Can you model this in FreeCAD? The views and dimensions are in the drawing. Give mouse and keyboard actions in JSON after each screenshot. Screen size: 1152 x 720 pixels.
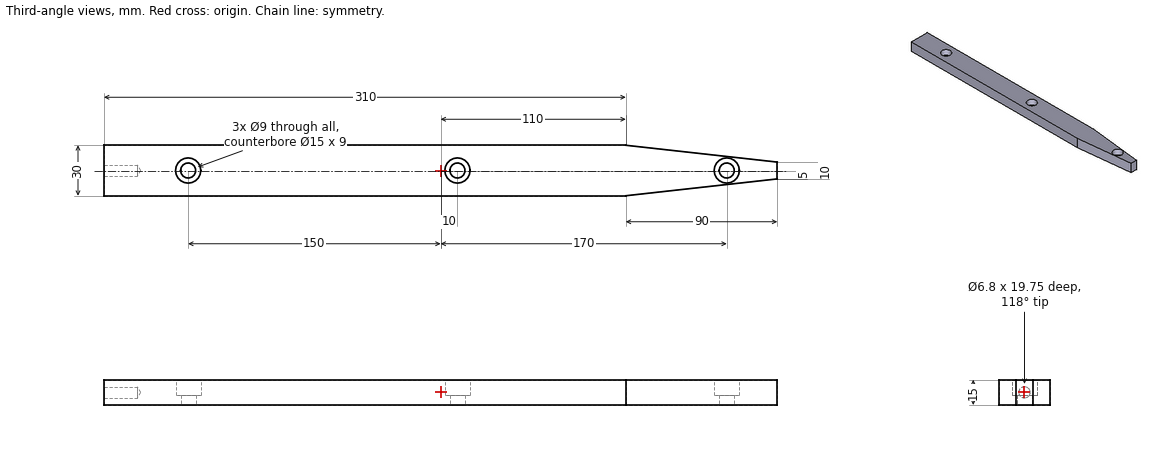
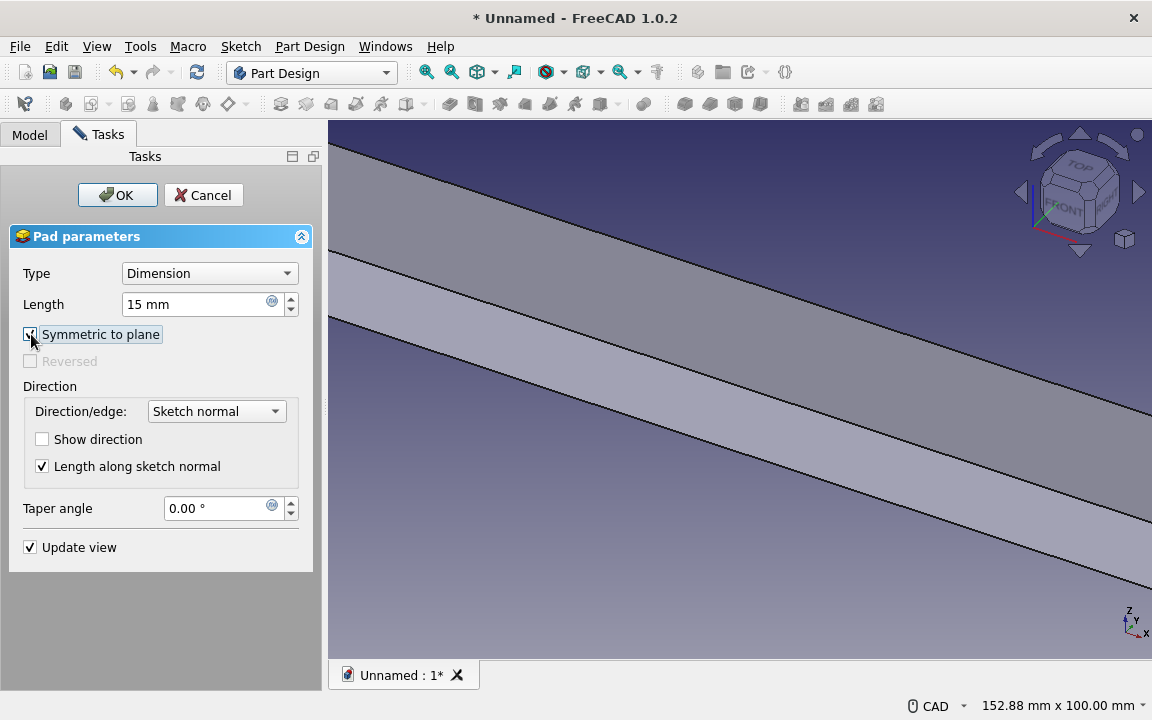
{"action": "left_click", "coordinate": [118, 195]}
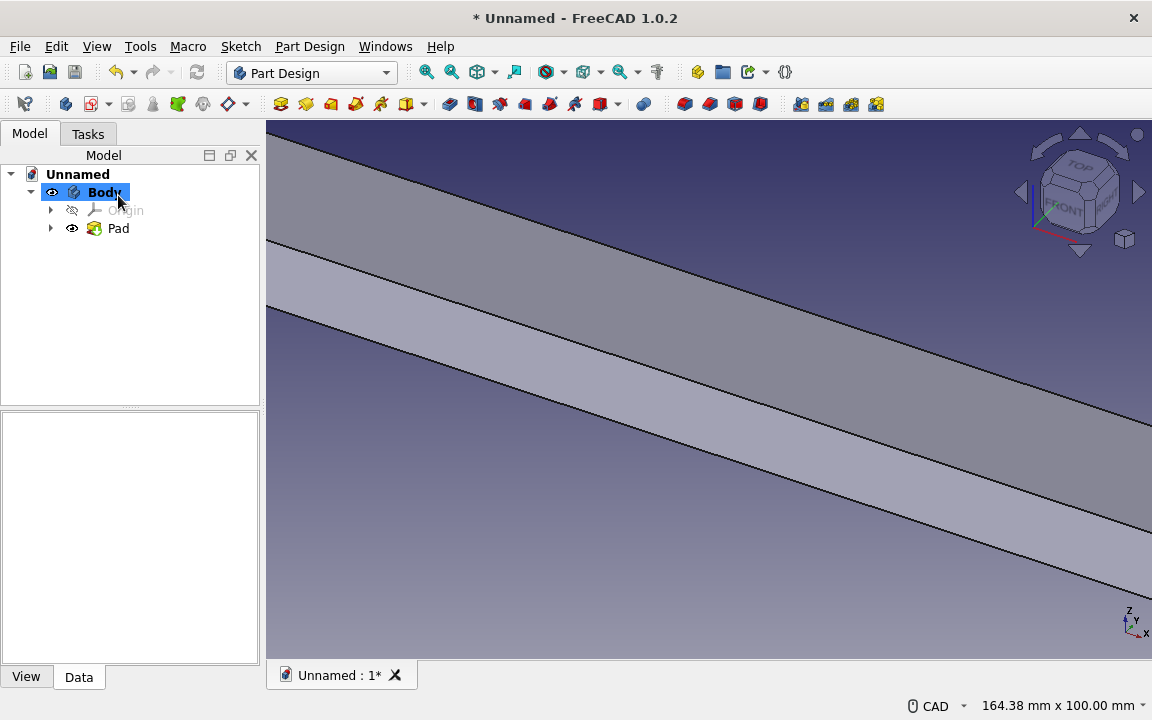
{"action": "key", "text": "v f"}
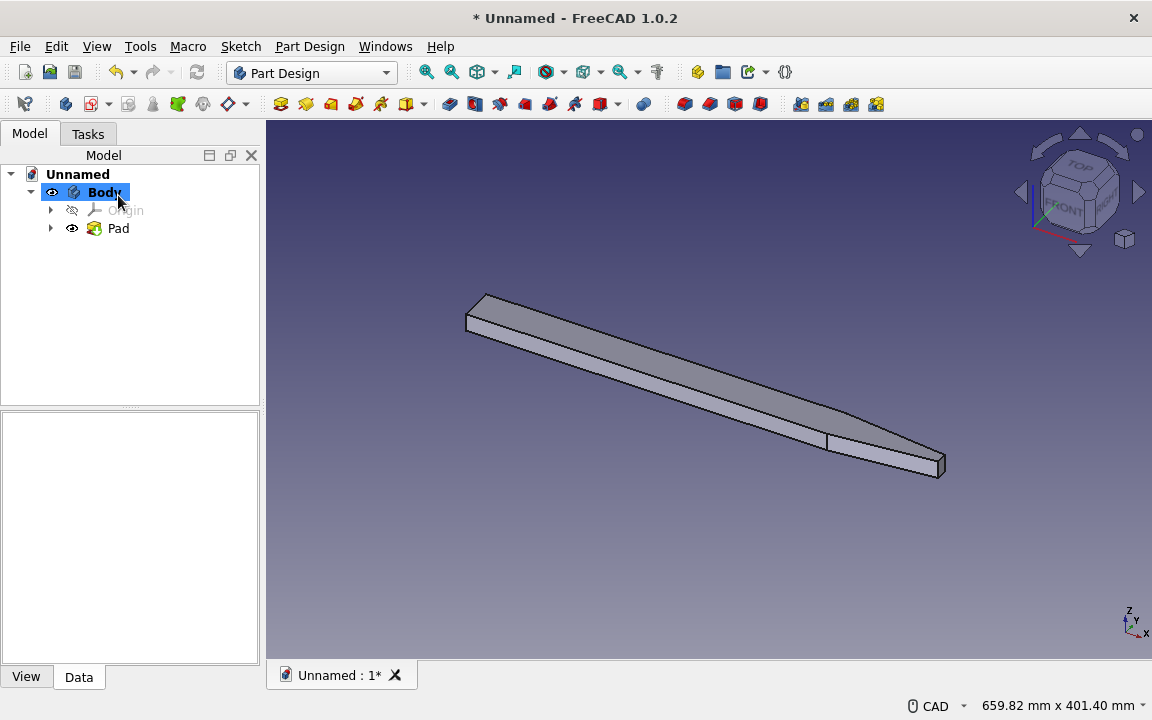
{"action": "key", "text": "6"}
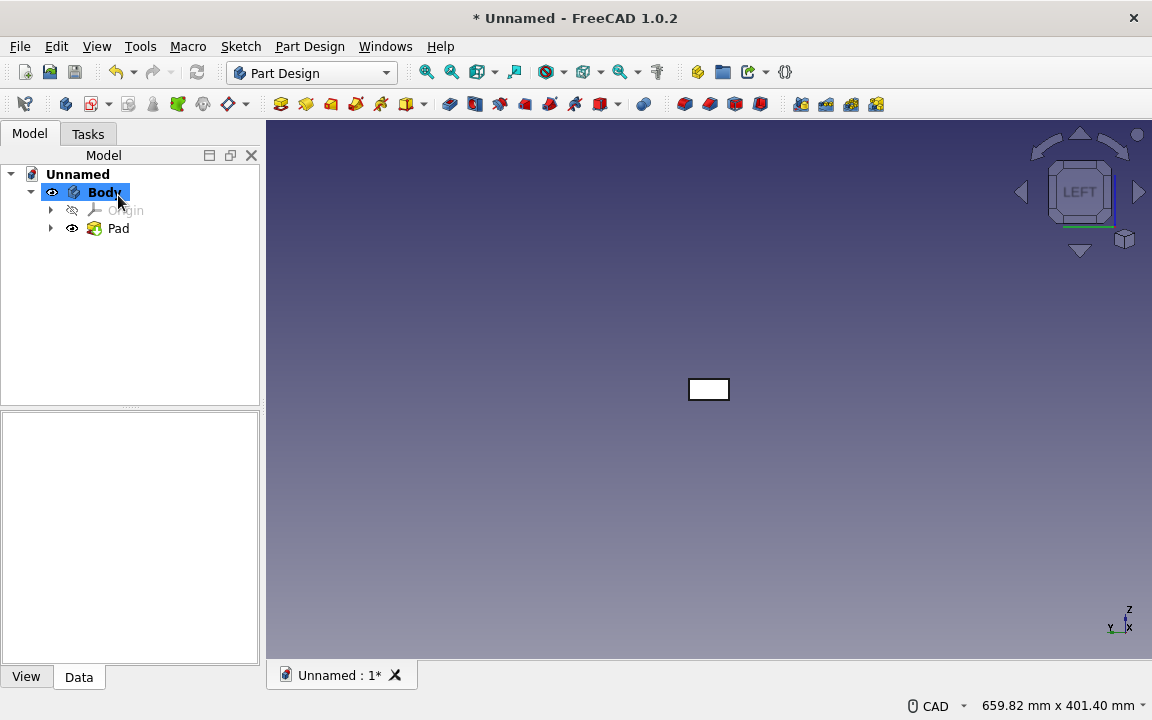
{"action": "key", "text": "v f"}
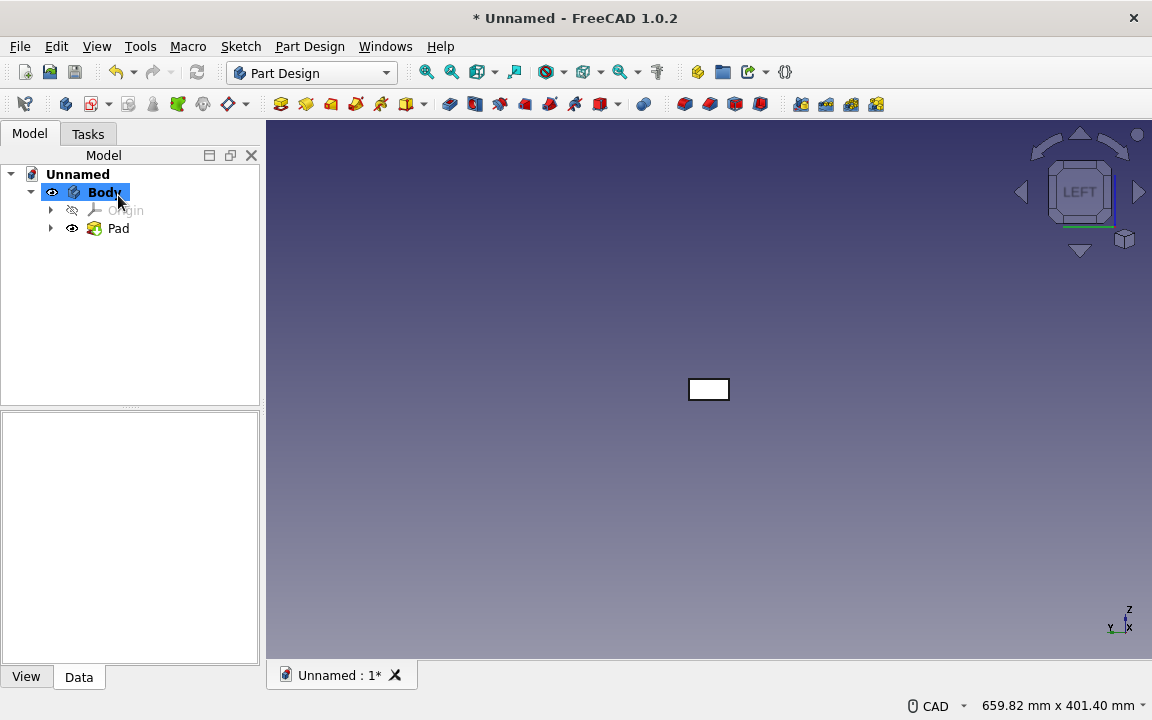
{"action": "left_click", "coordinate": [703, 388]}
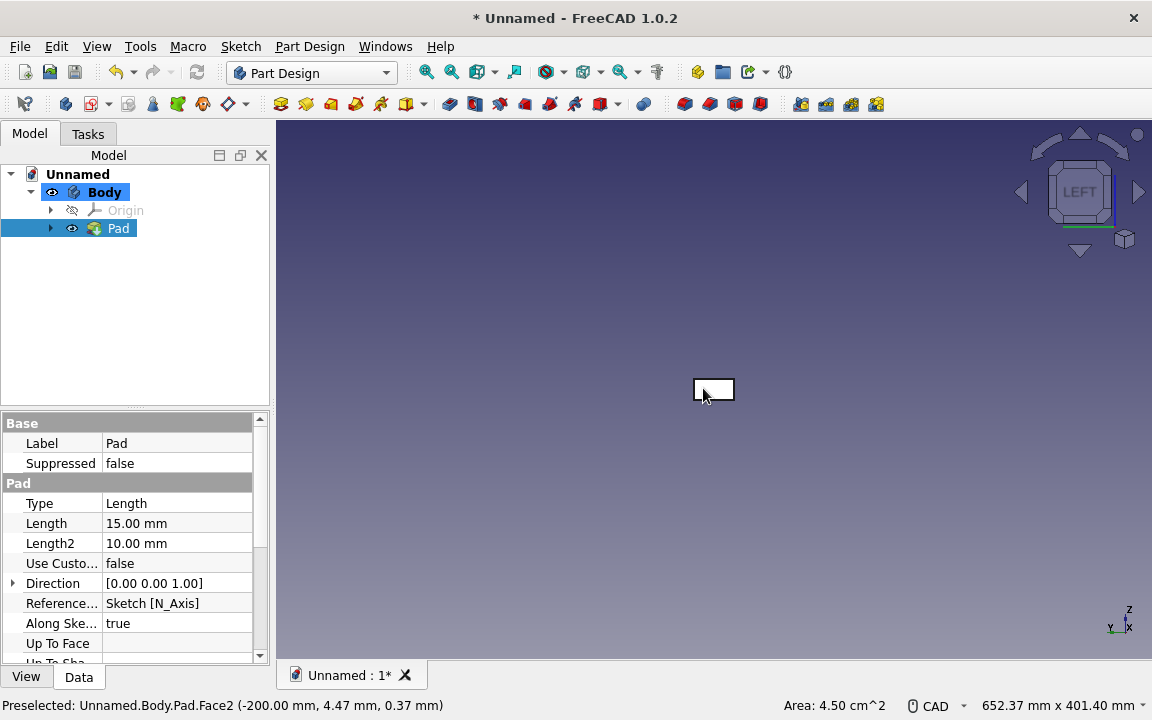
{"action": "left_click", "coordinate": [90, 104]}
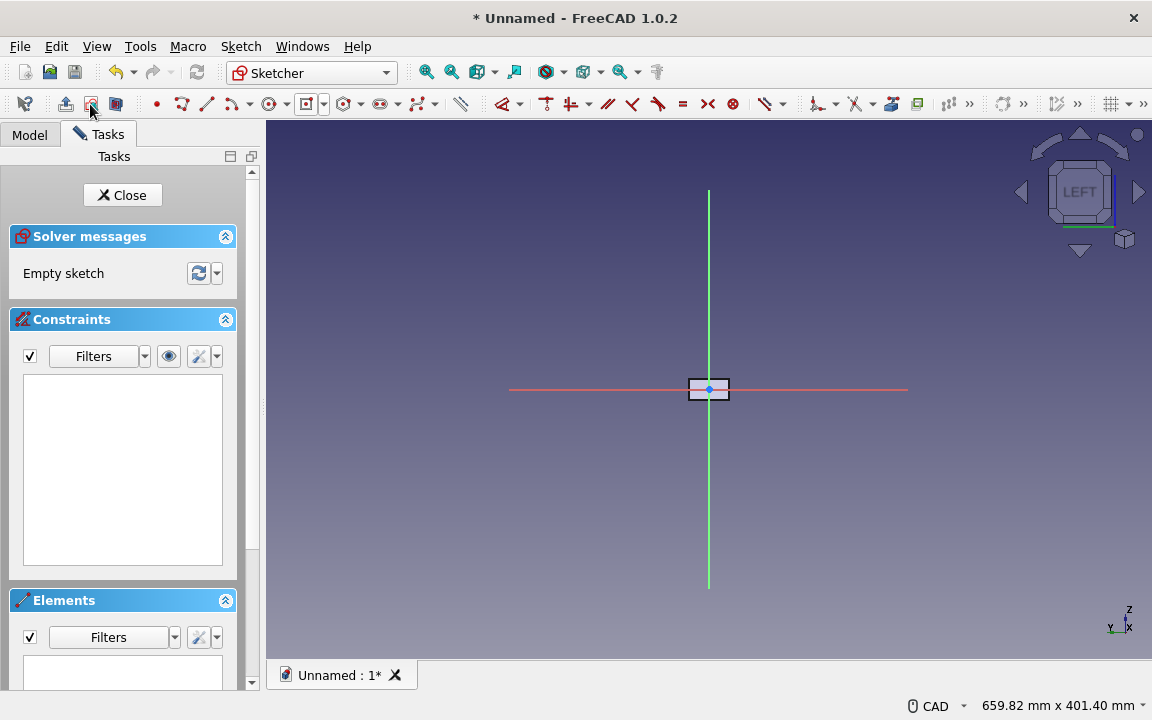
{"action": "scroll", "coordinate": [713, 390], "scroll_direction": "up", "scroll_amount": 15}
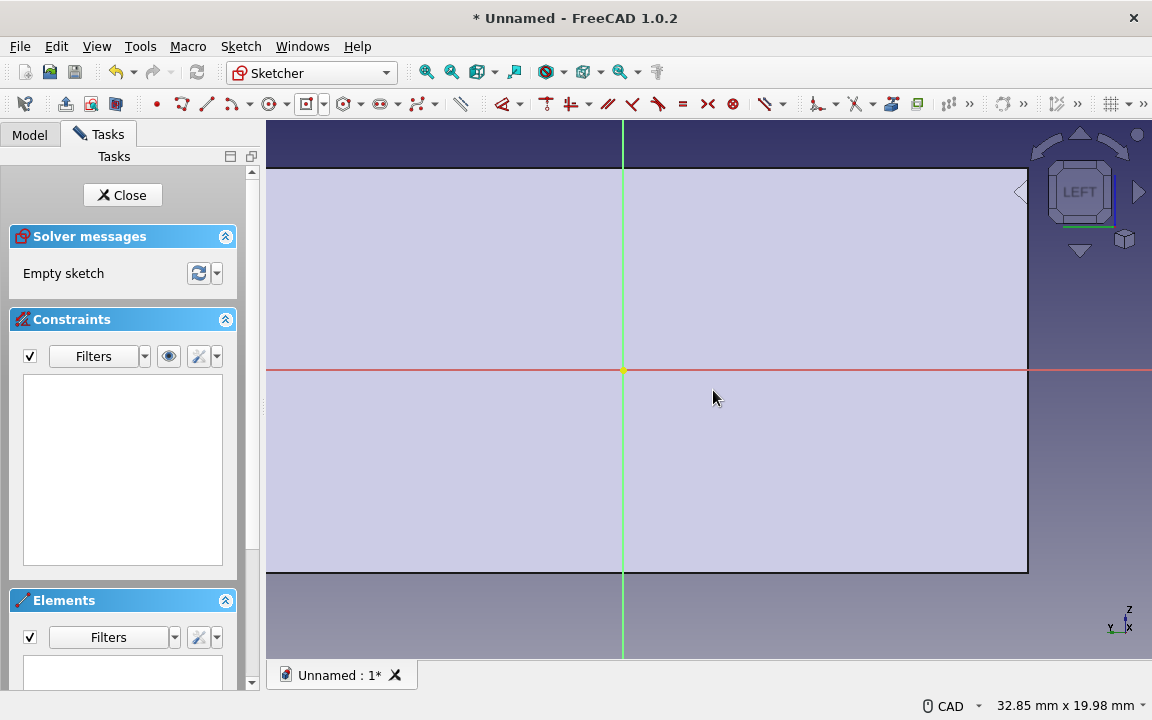
{"action": "scroll", "coordinate": [602, 347], "scroll_direction": "up", "scroll_amount": 3}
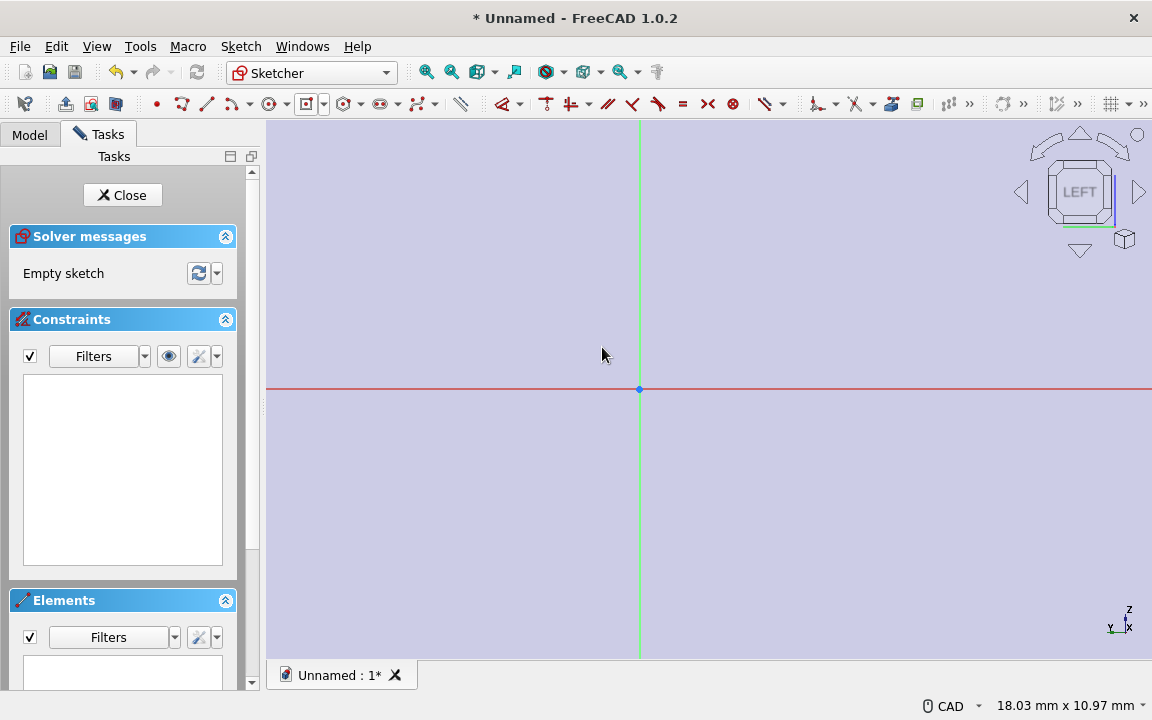
{"action": "left_click", "coordinate": [268, 104]}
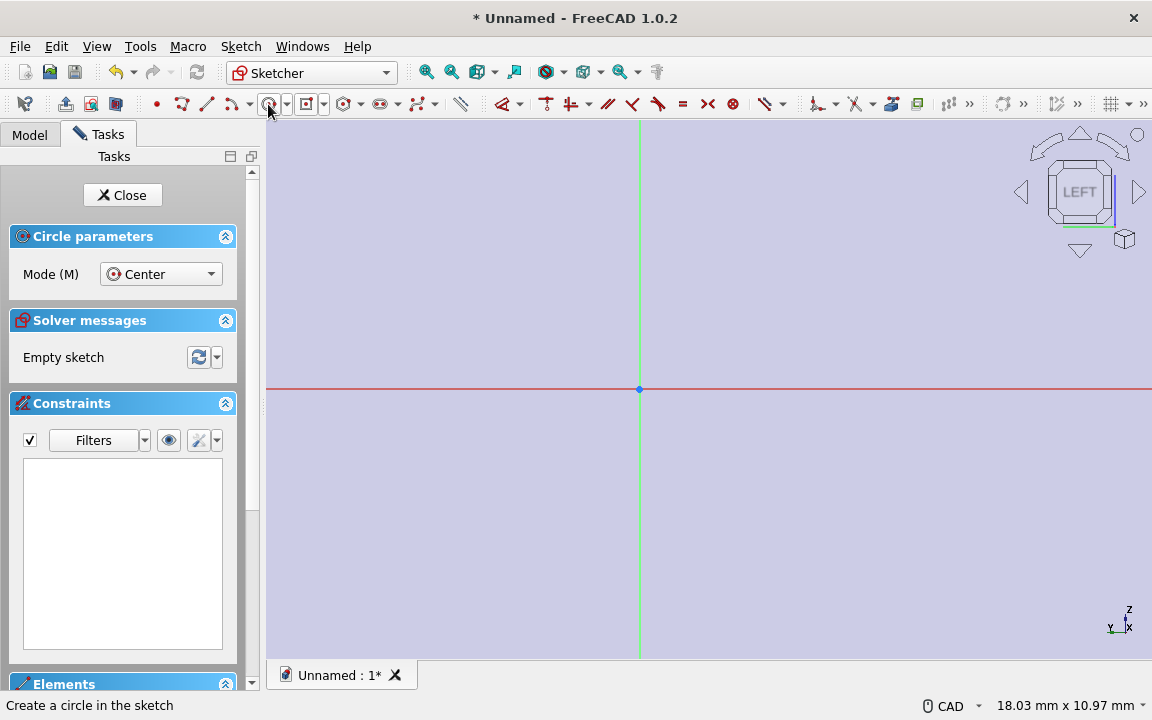
{"action": "left_click", "coordinate": [640, 389]}
{"action": "mouse_move", "coordinate": [758, 271]}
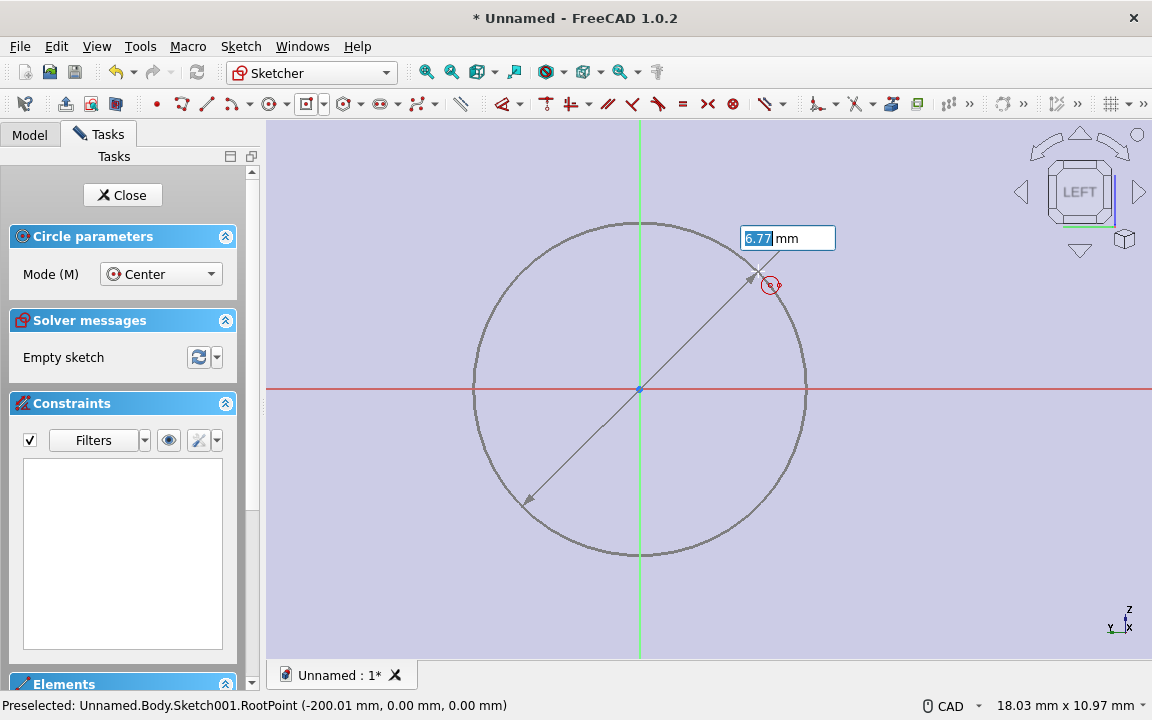
{"action": "type", "text": "6.8"}
{"action": "key", "text": "Return"}
{"action": "key", "text": "Escape"}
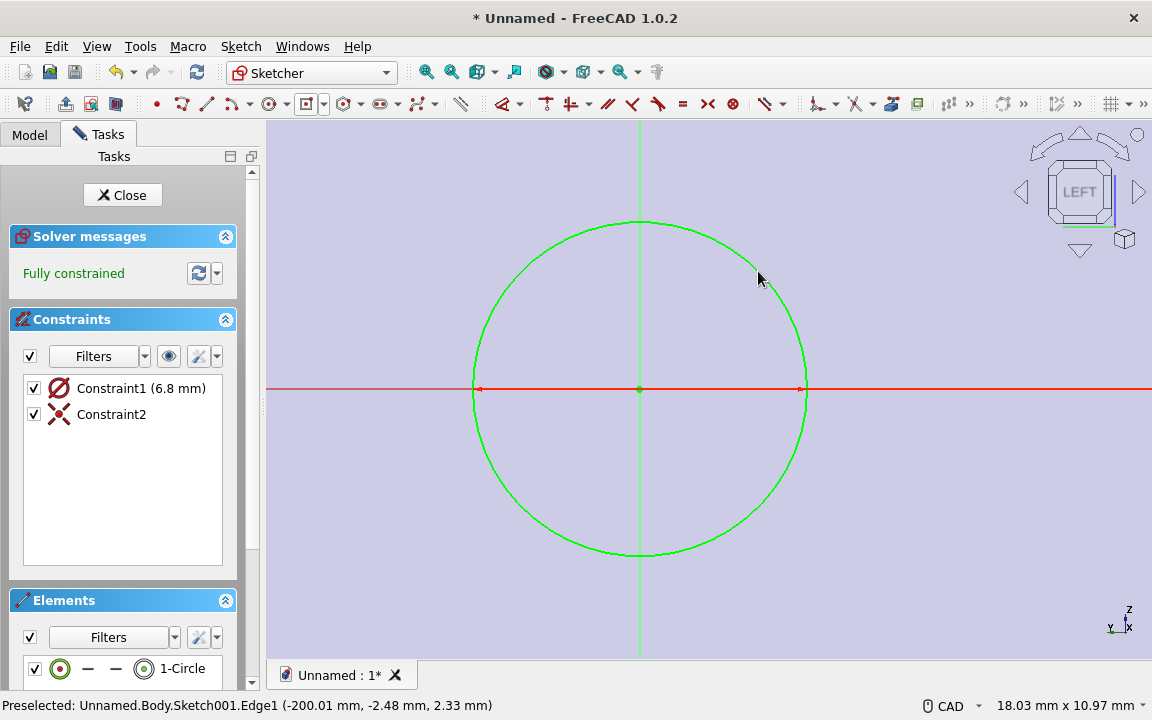
{"action": "left_click", "coordinate": [123, 195]}